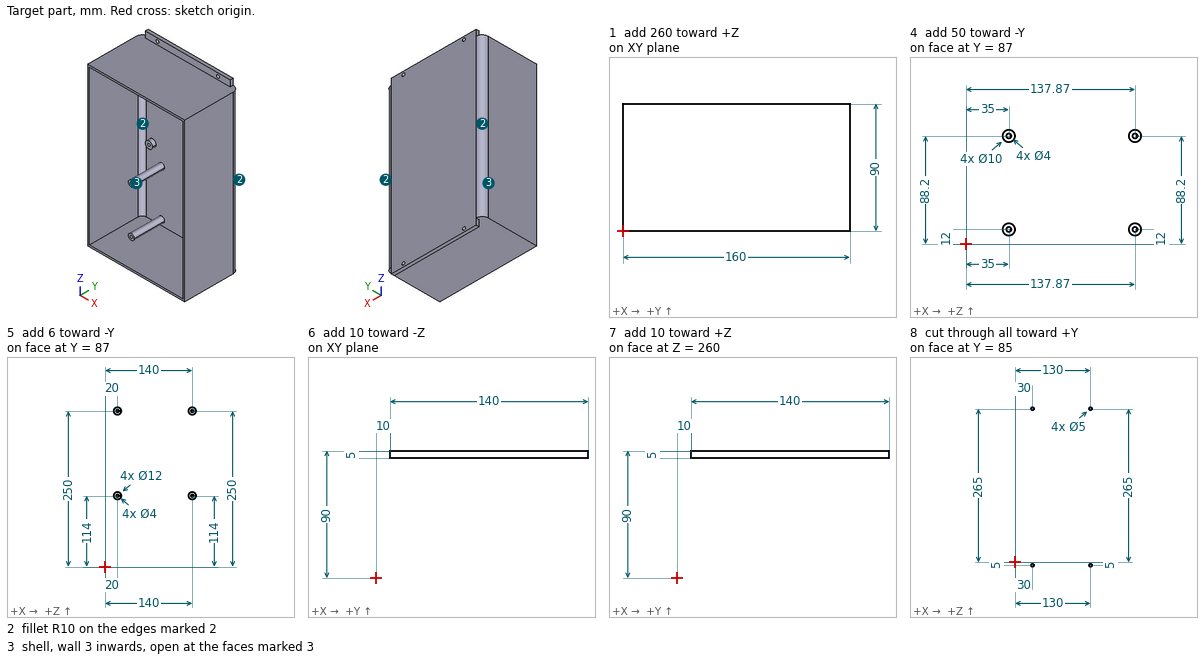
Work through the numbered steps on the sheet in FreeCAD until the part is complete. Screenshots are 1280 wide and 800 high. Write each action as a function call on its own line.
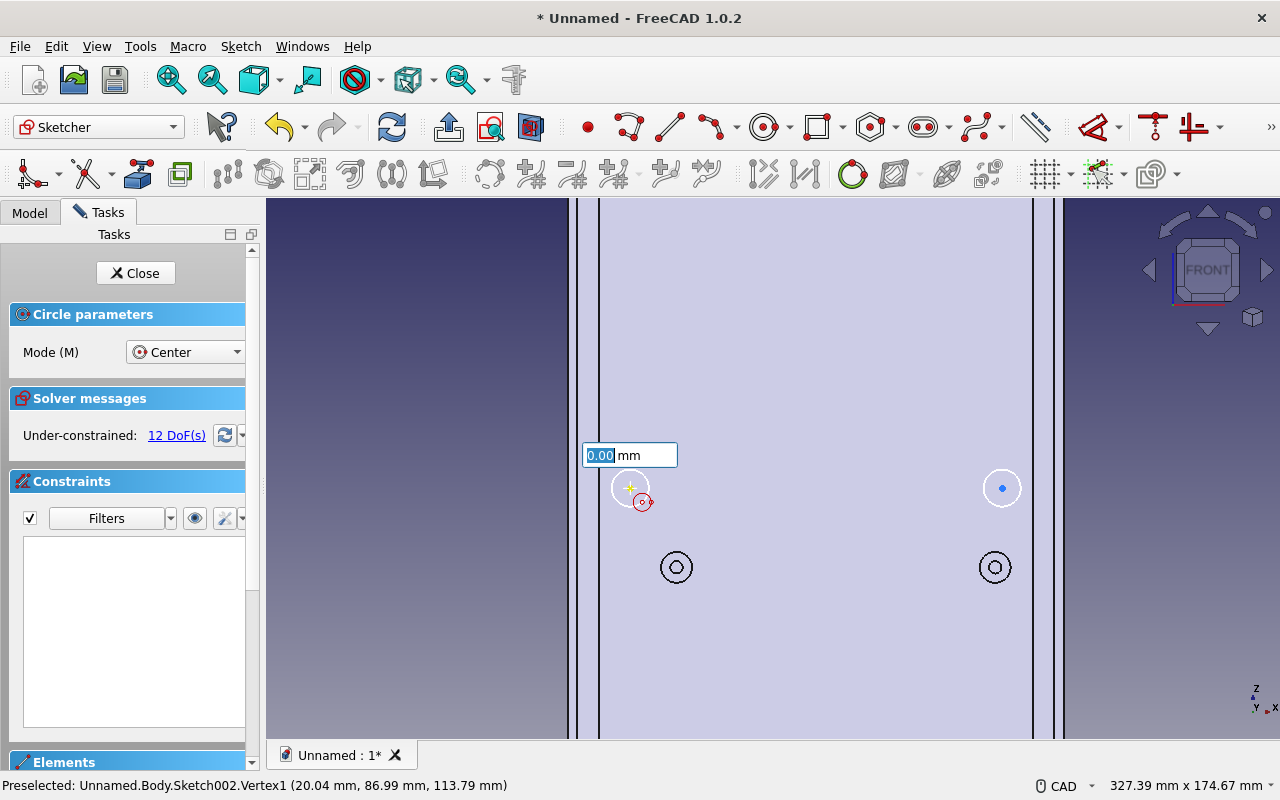
scroll(636, 485, up, 5)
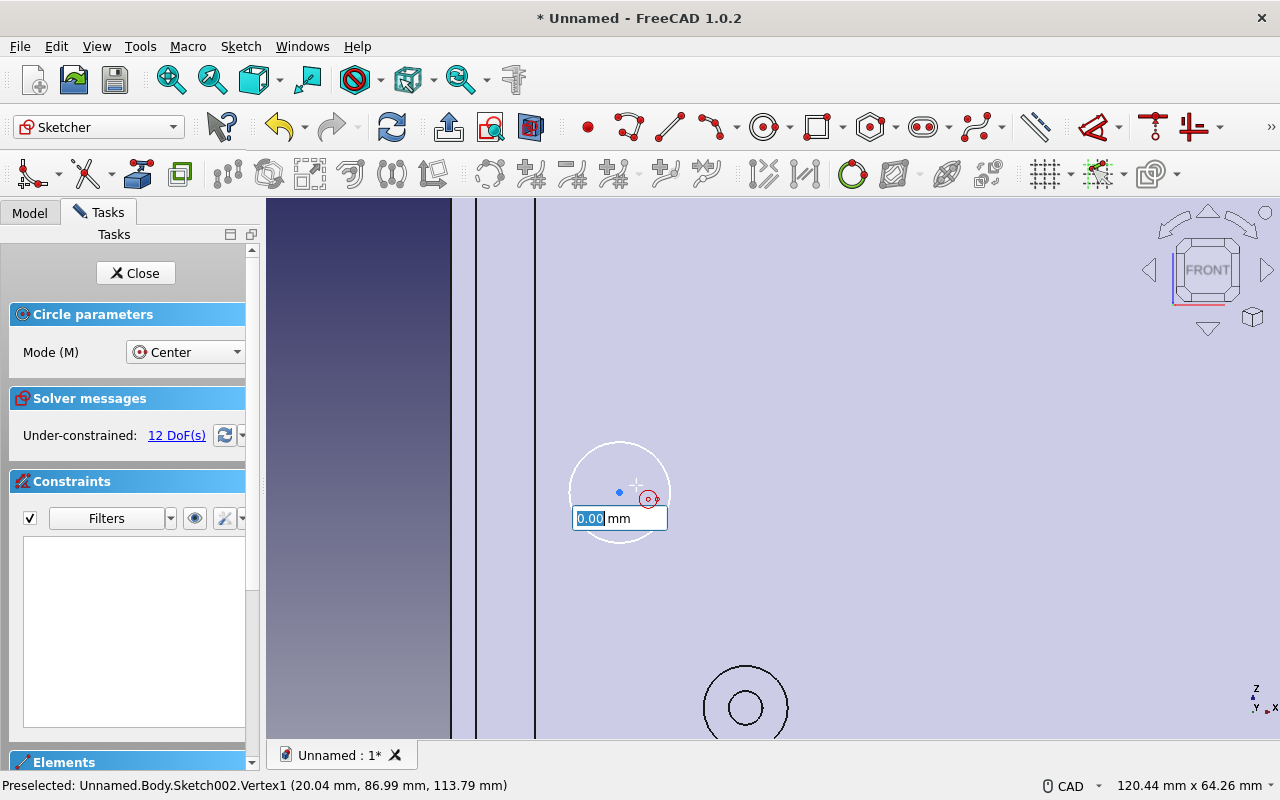
click(635, 485)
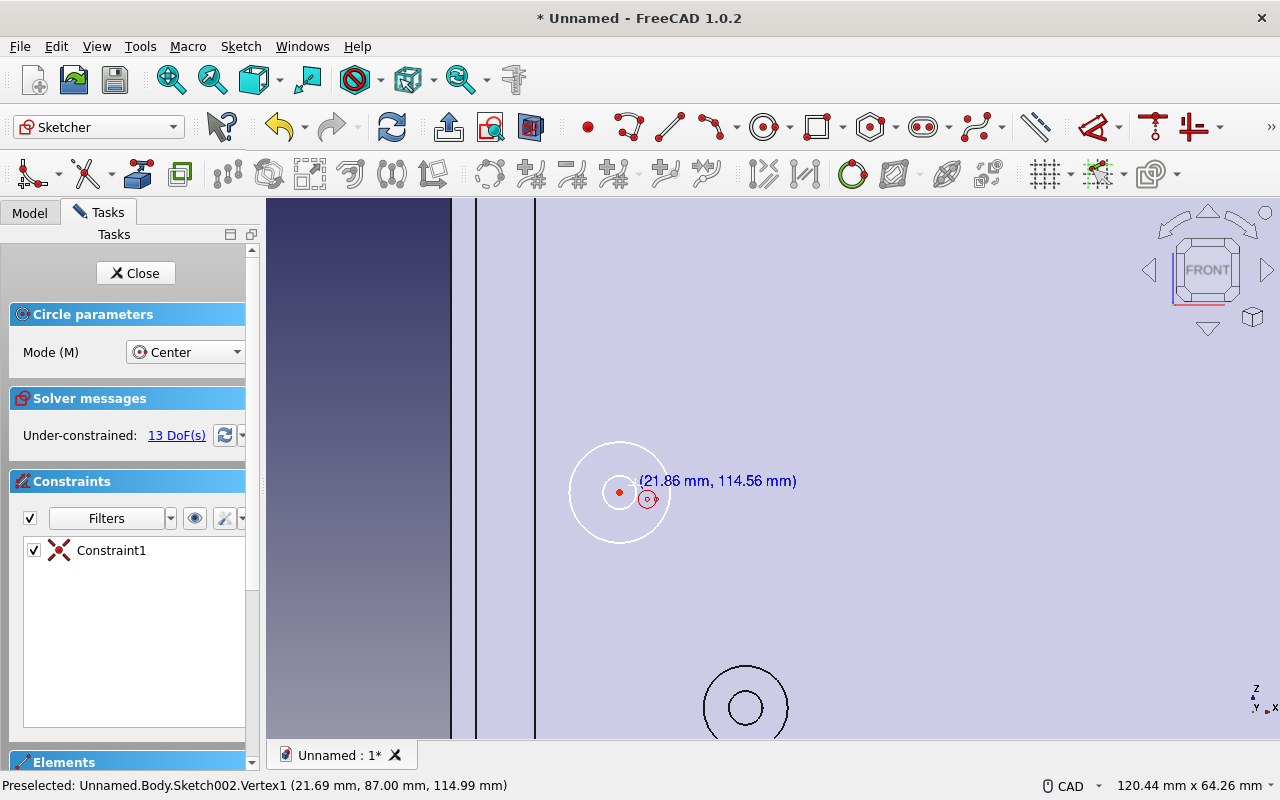
scroll(633, 487, down, 9)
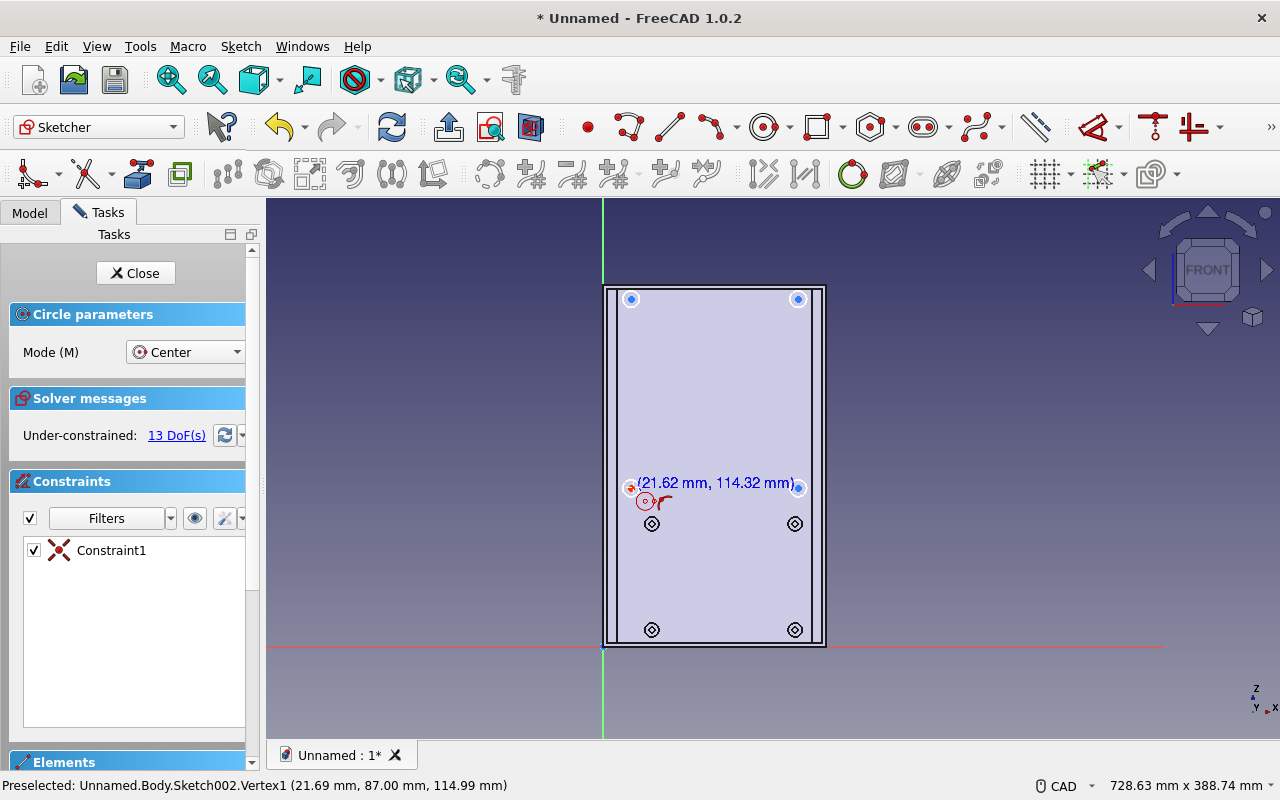
scroll(631, 299, up, 11)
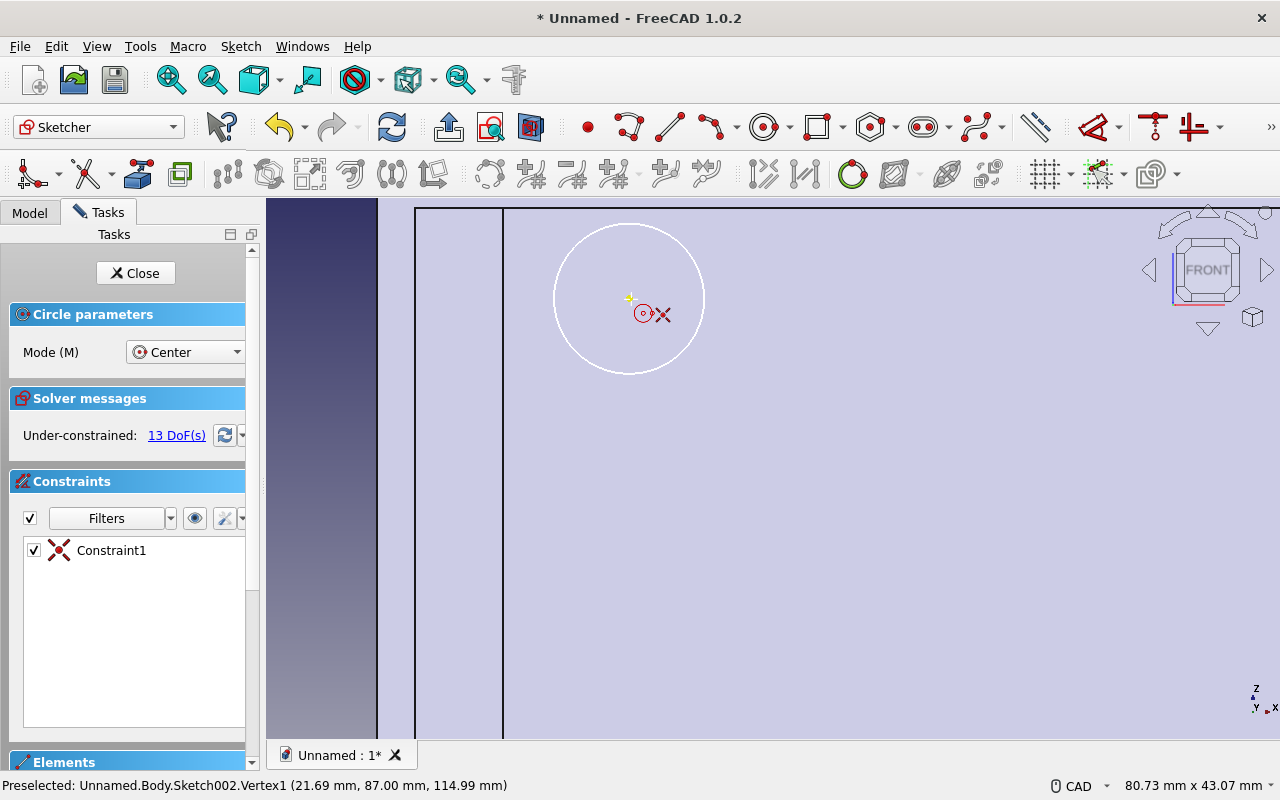
scroll(631, 299, down, 11)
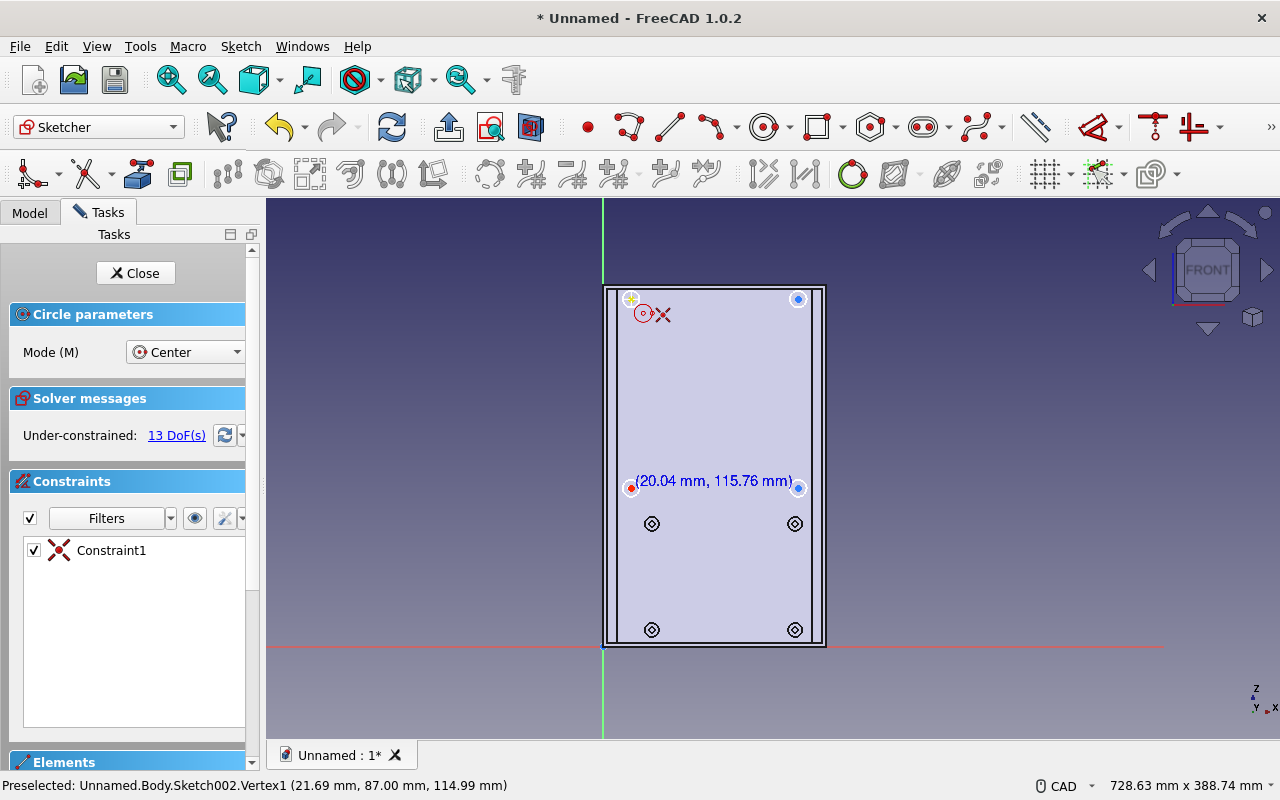
scroll(631, 299, up, 4)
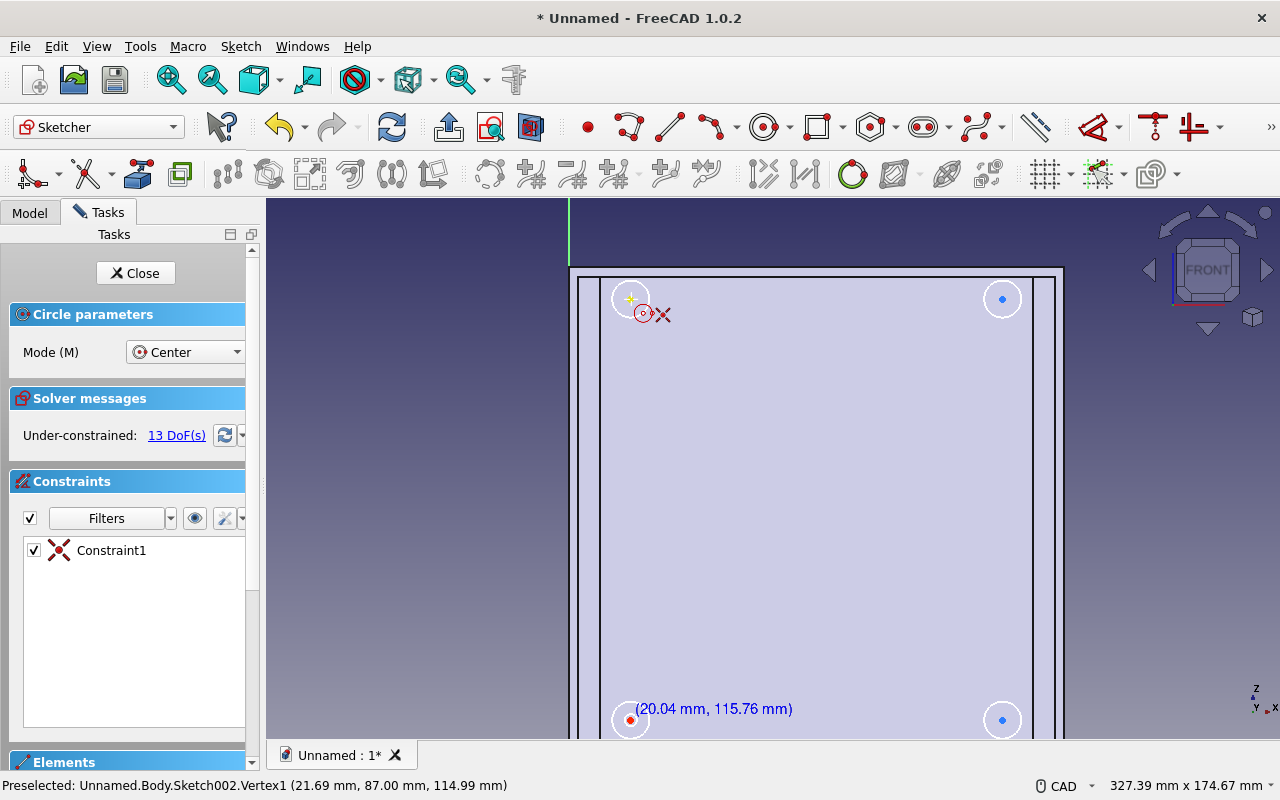
click(631, 299)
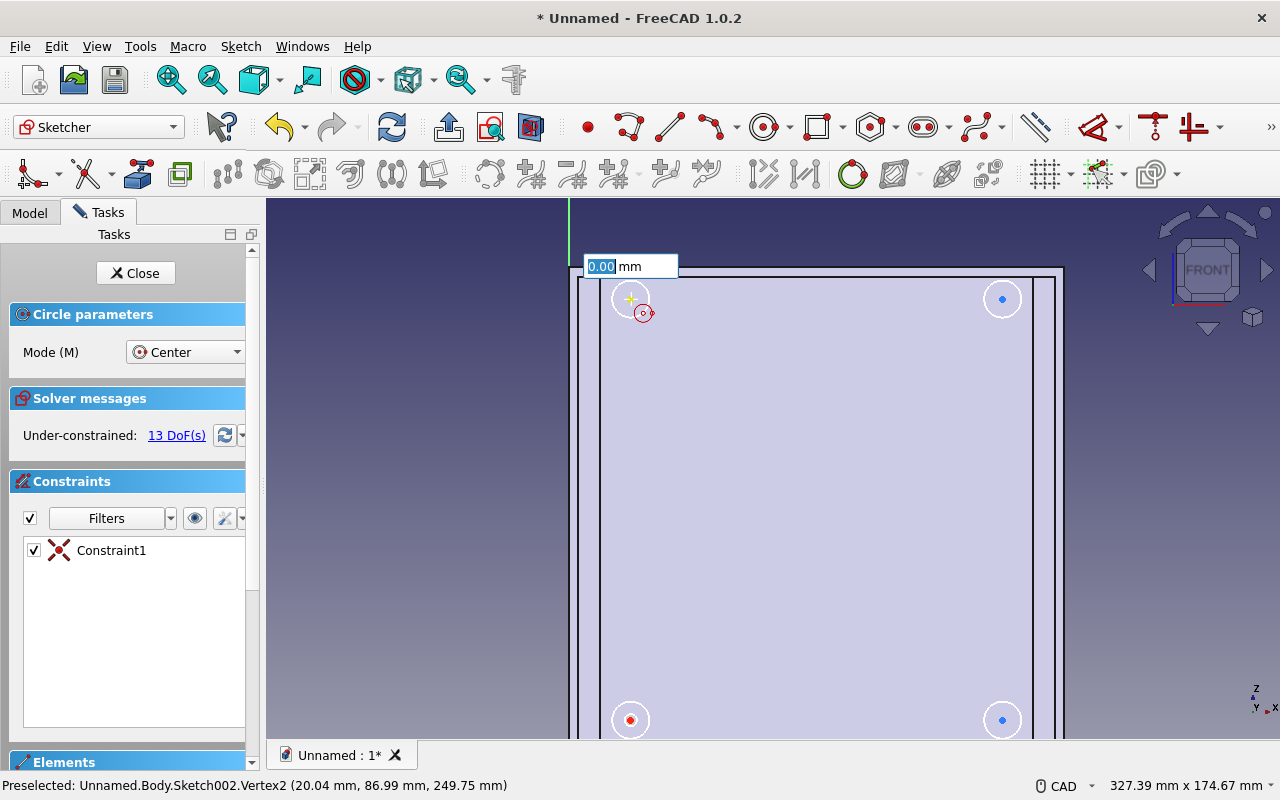
scroll(635, 294, up, 5)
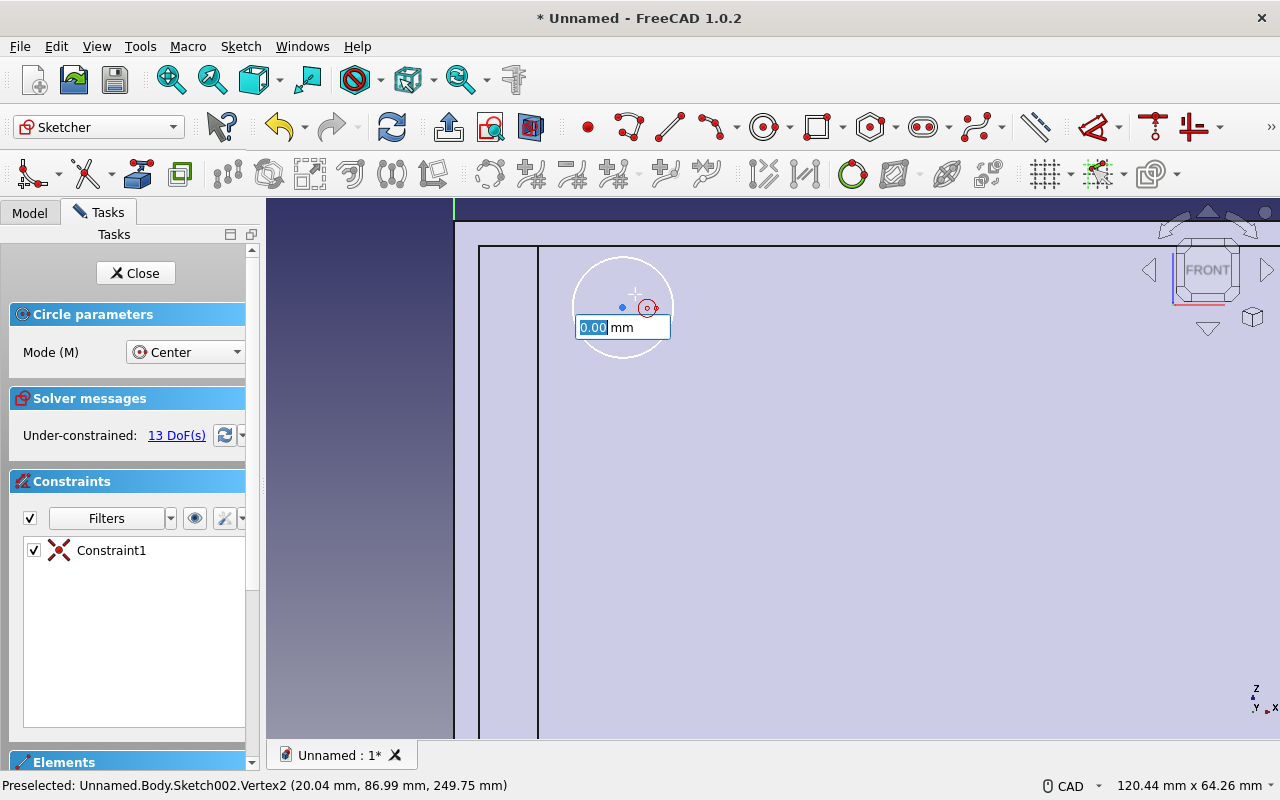
click(635, 294)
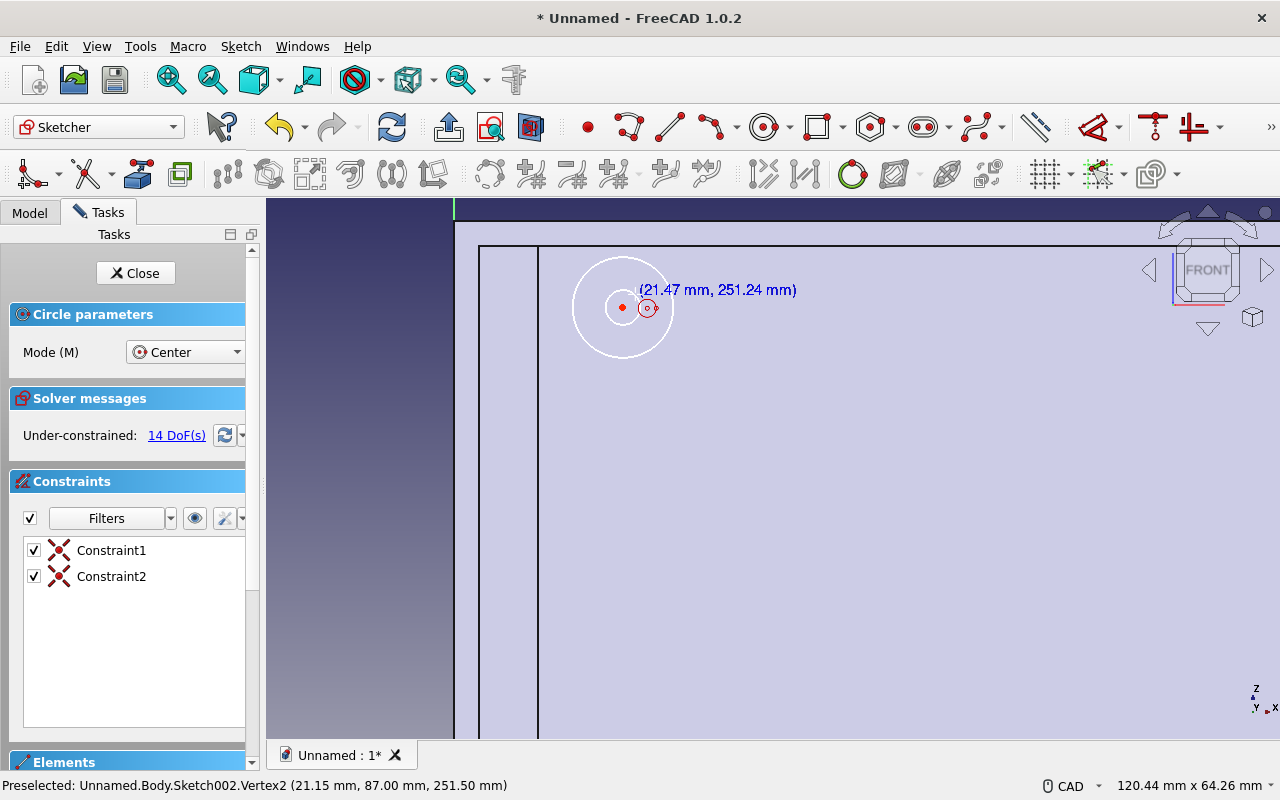
scroll(632, 297, down, 9)